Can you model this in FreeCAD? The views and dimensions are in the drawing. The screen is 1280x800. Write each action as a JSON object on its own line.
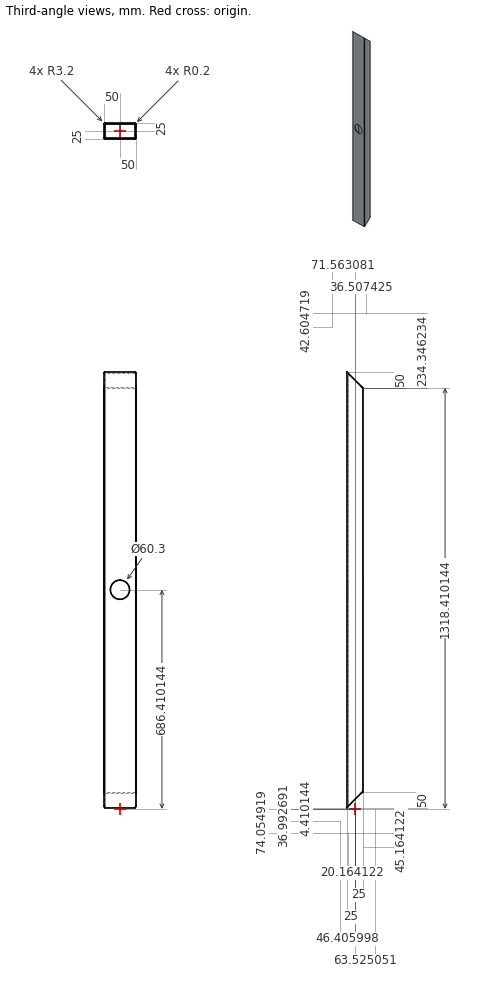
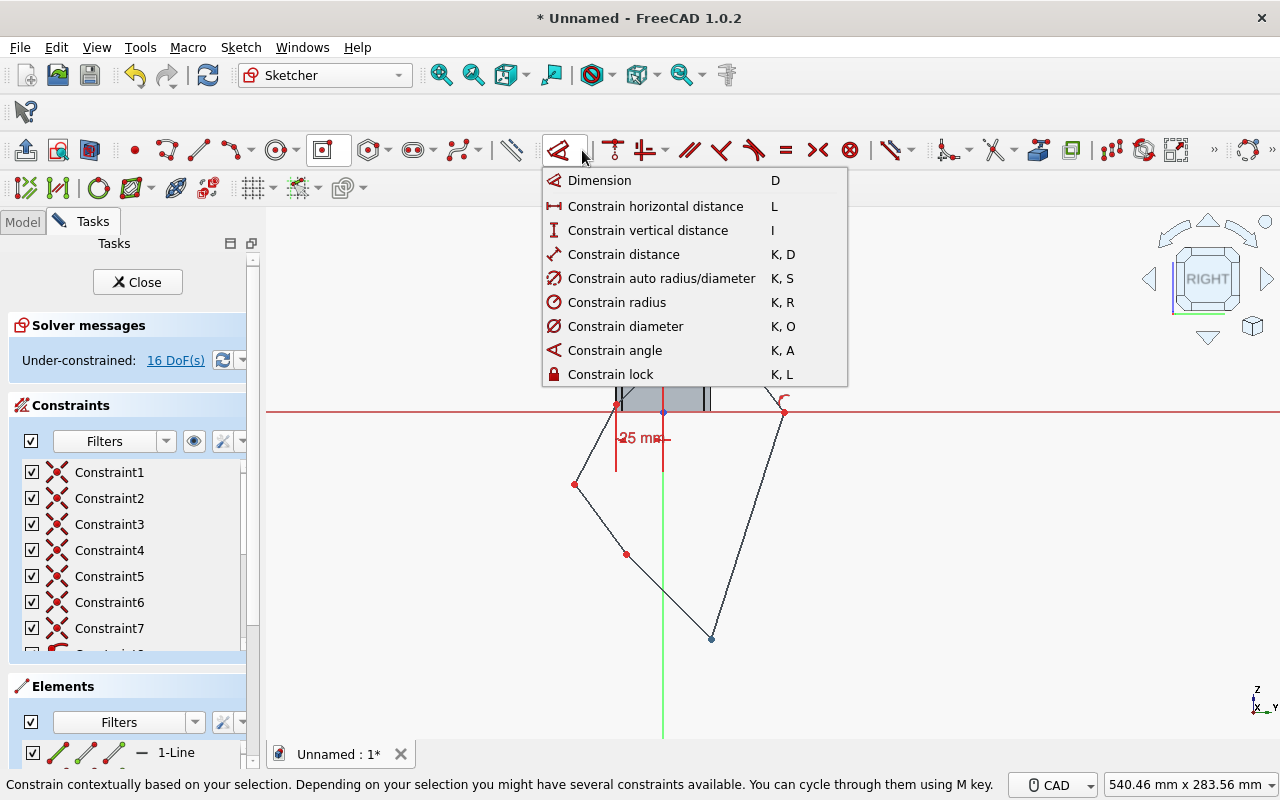
{"action": "left_click", "coordinate": [695, 206]}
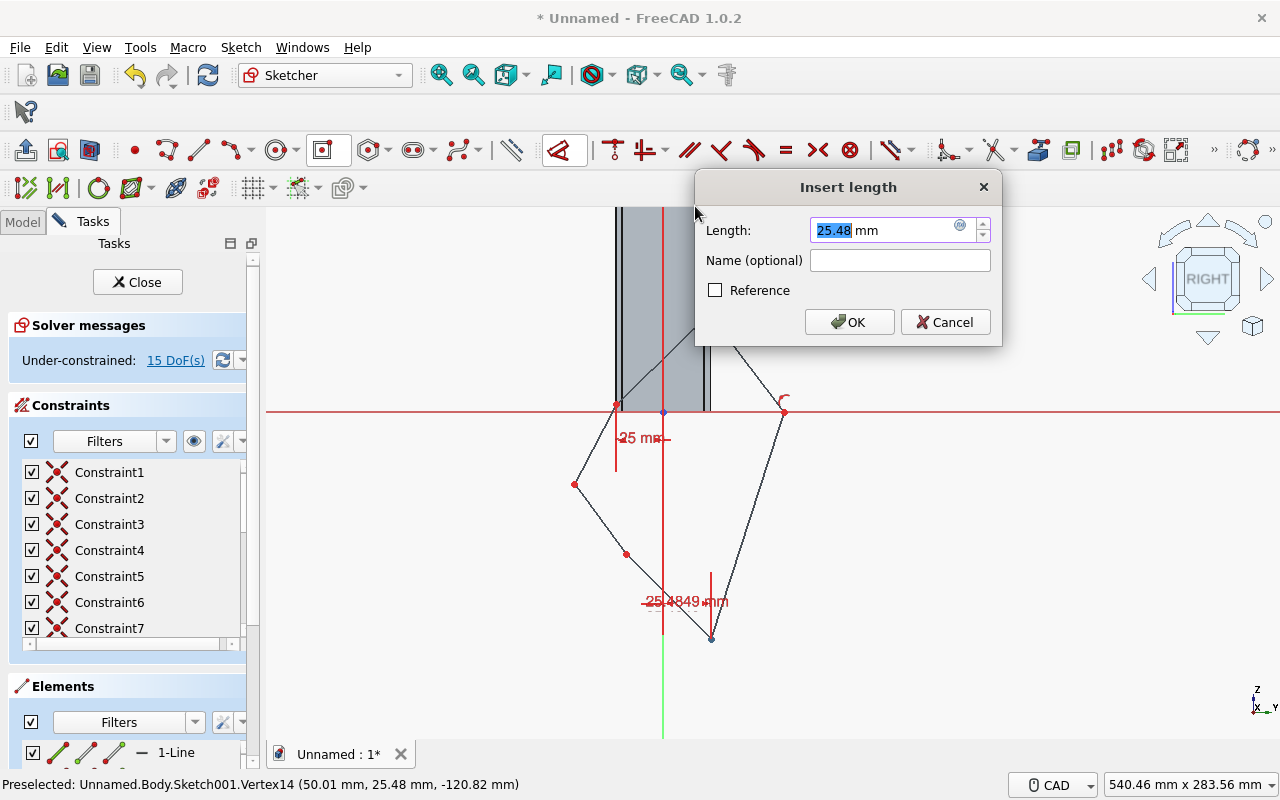
{"action": "type", "text": "25"}
{"action": "key", "text": "Return"}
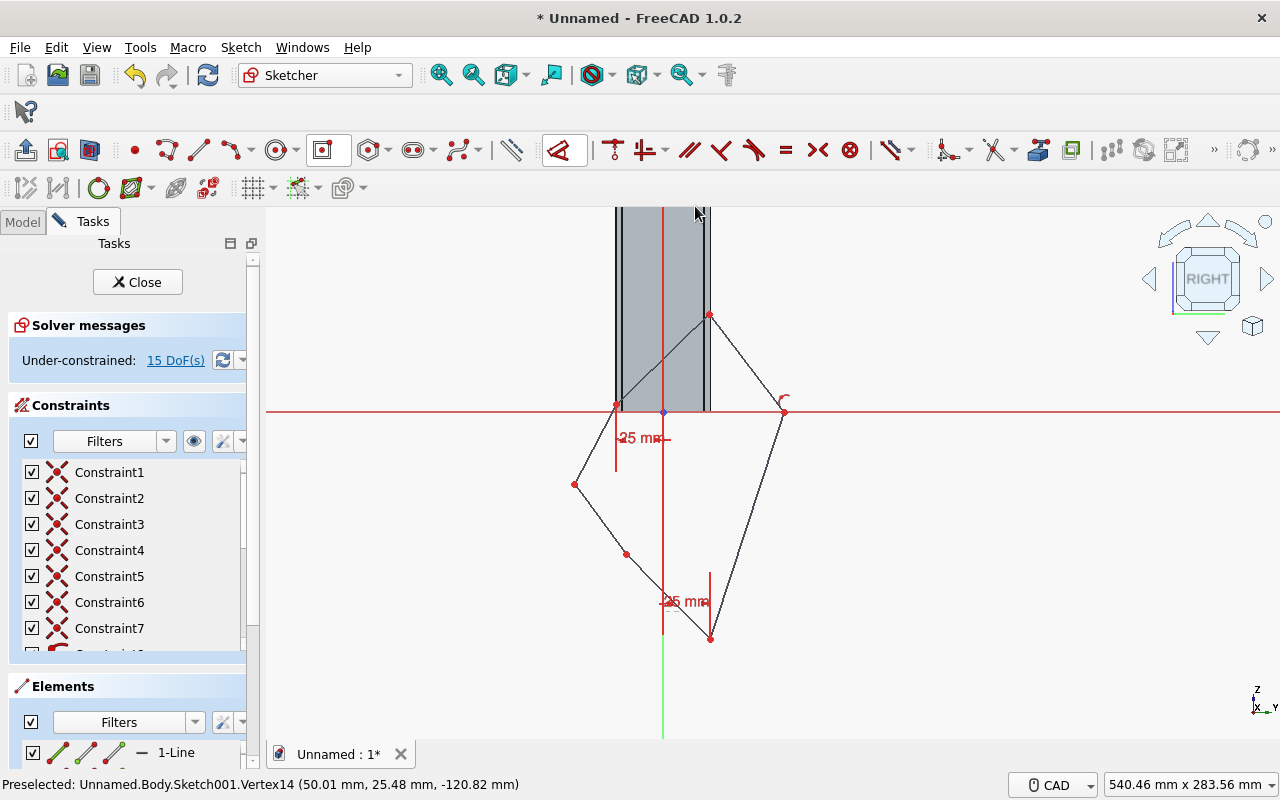
{"action": "left_click", "coordinate": [709, 314]}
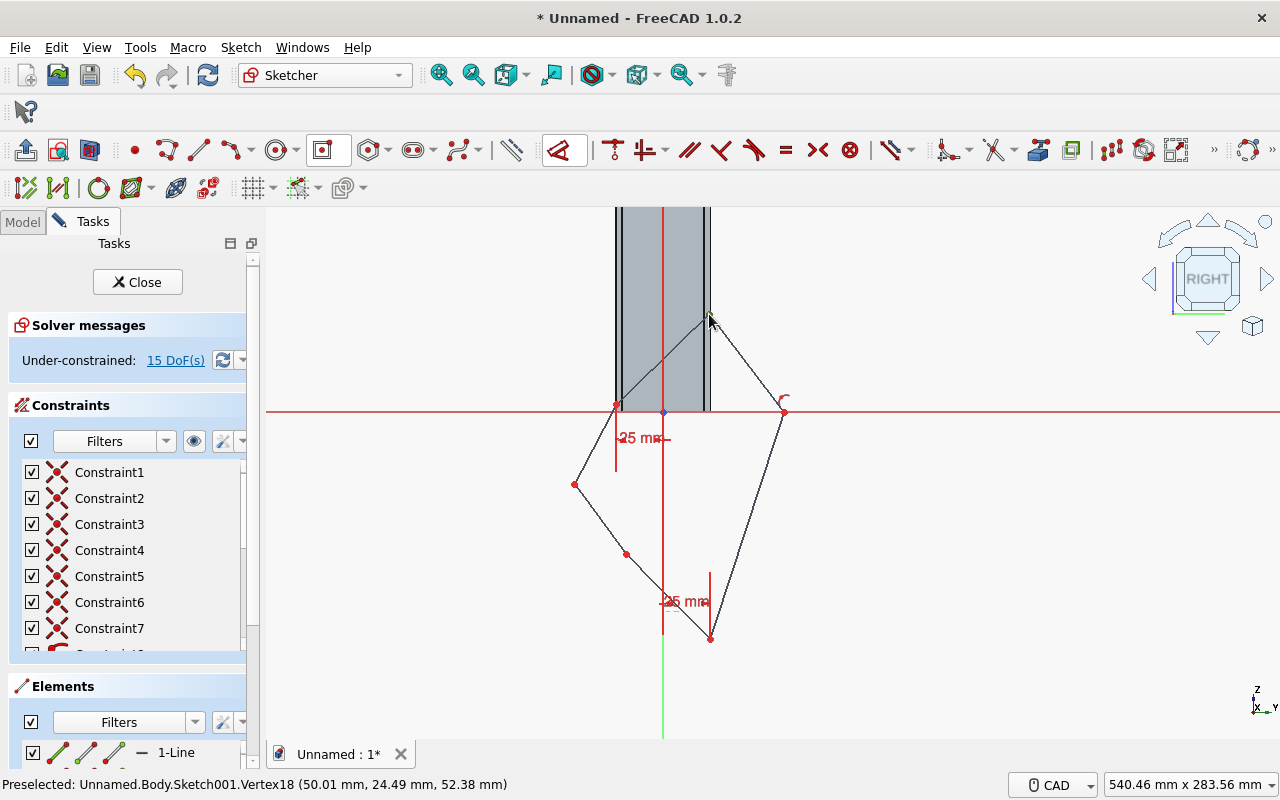
{"action": "left_click", "coordinate": [582, 150]}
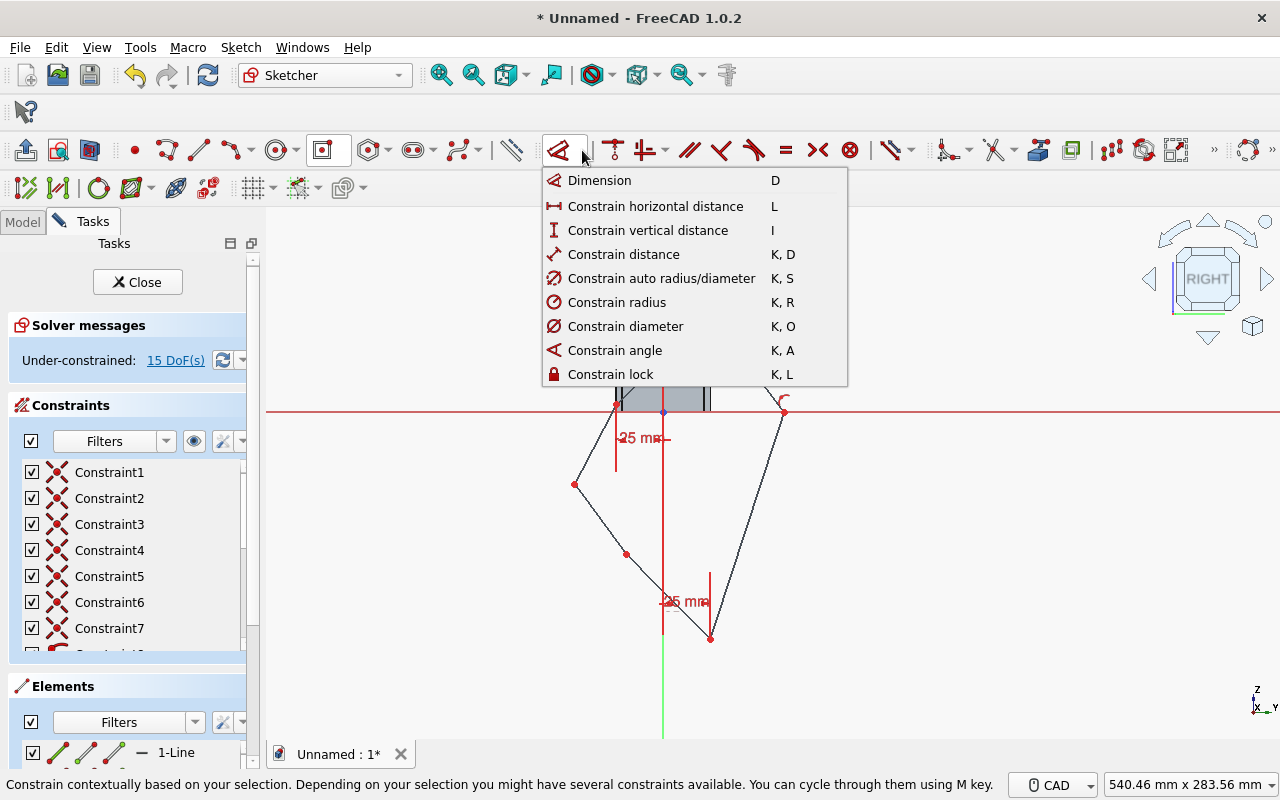
{"action": "left_click", "coordinate": [695, 206]}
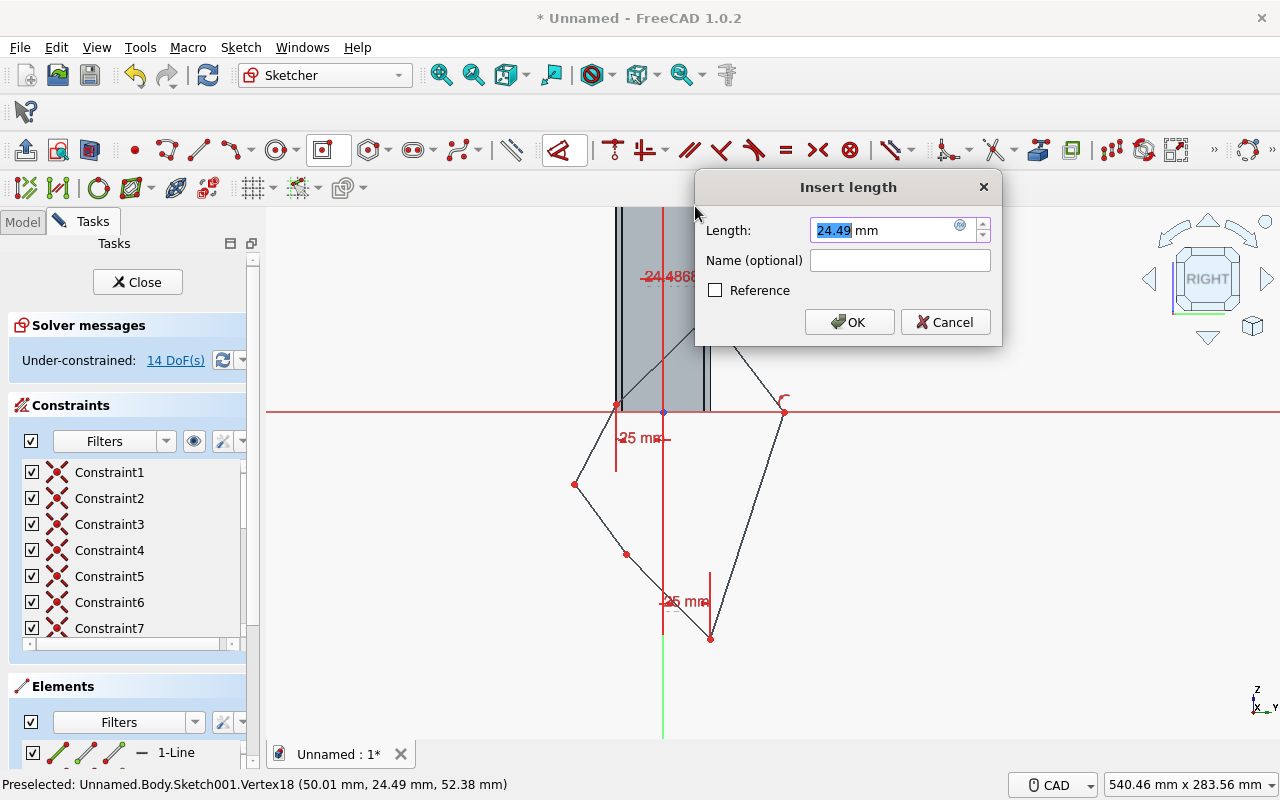
{"action": "type", "text": "25"}
{"action": "key", "text": "Return"}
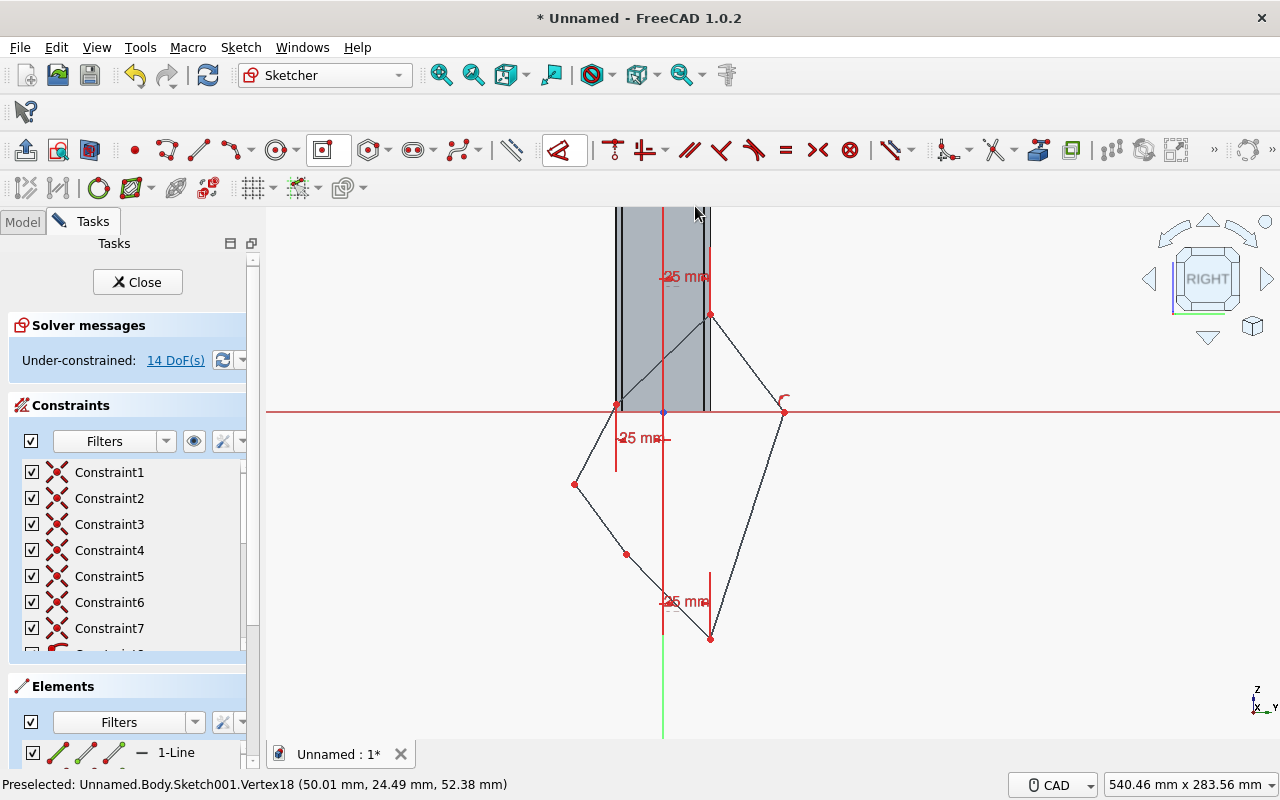
{"action": "scroll", "coordinate": [711, 648], "scroll_direction": "down", "scroll_amount": 11}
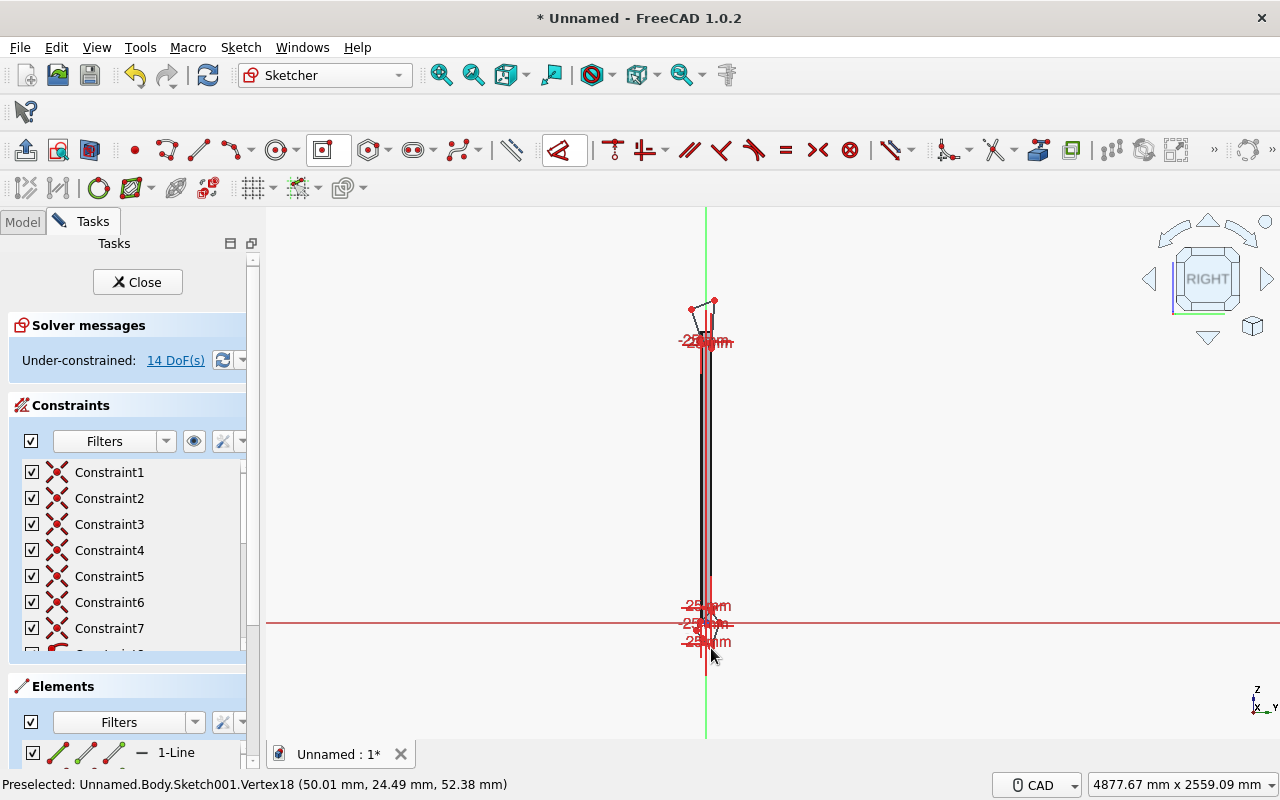
{"action": "scroll", "coordinate": [704, 342], "scroll_direction": "up", "scroll_amount": 10}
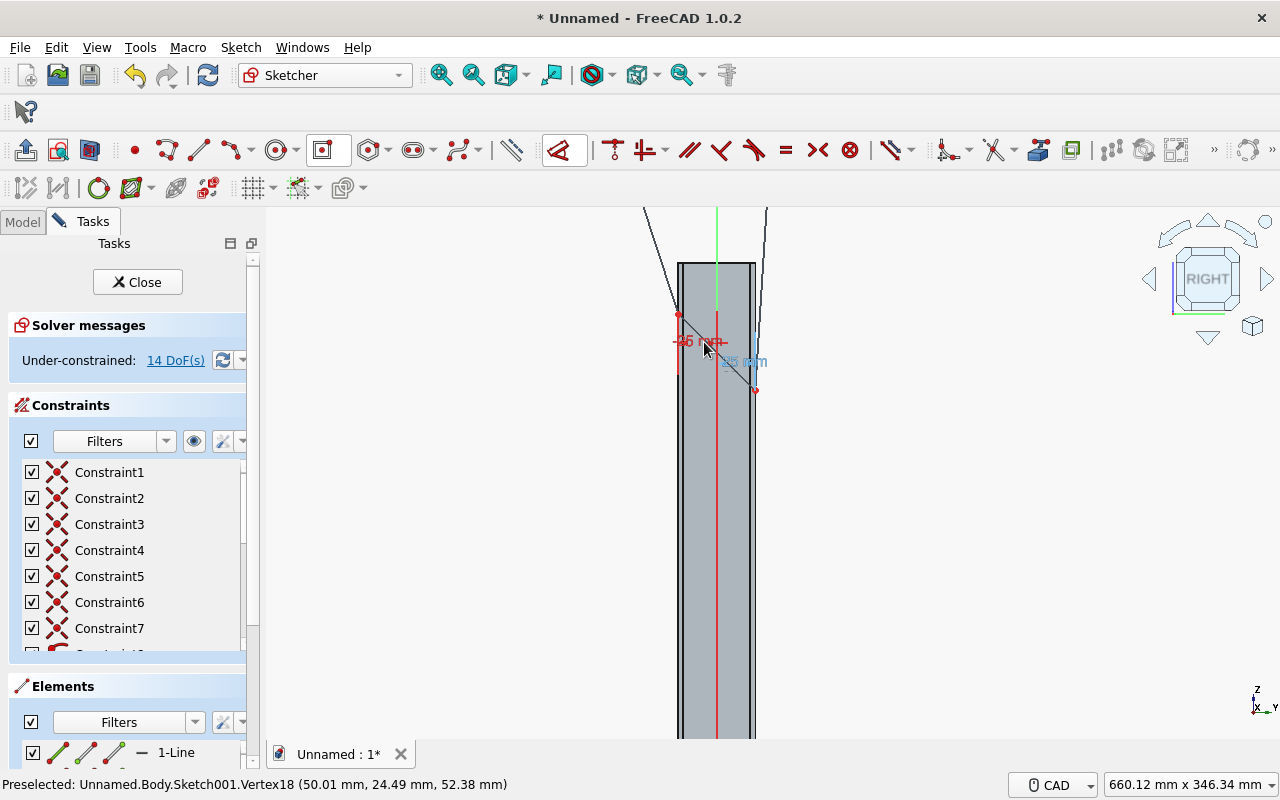
{"action": "left_click", "coordinate": [694, 329]}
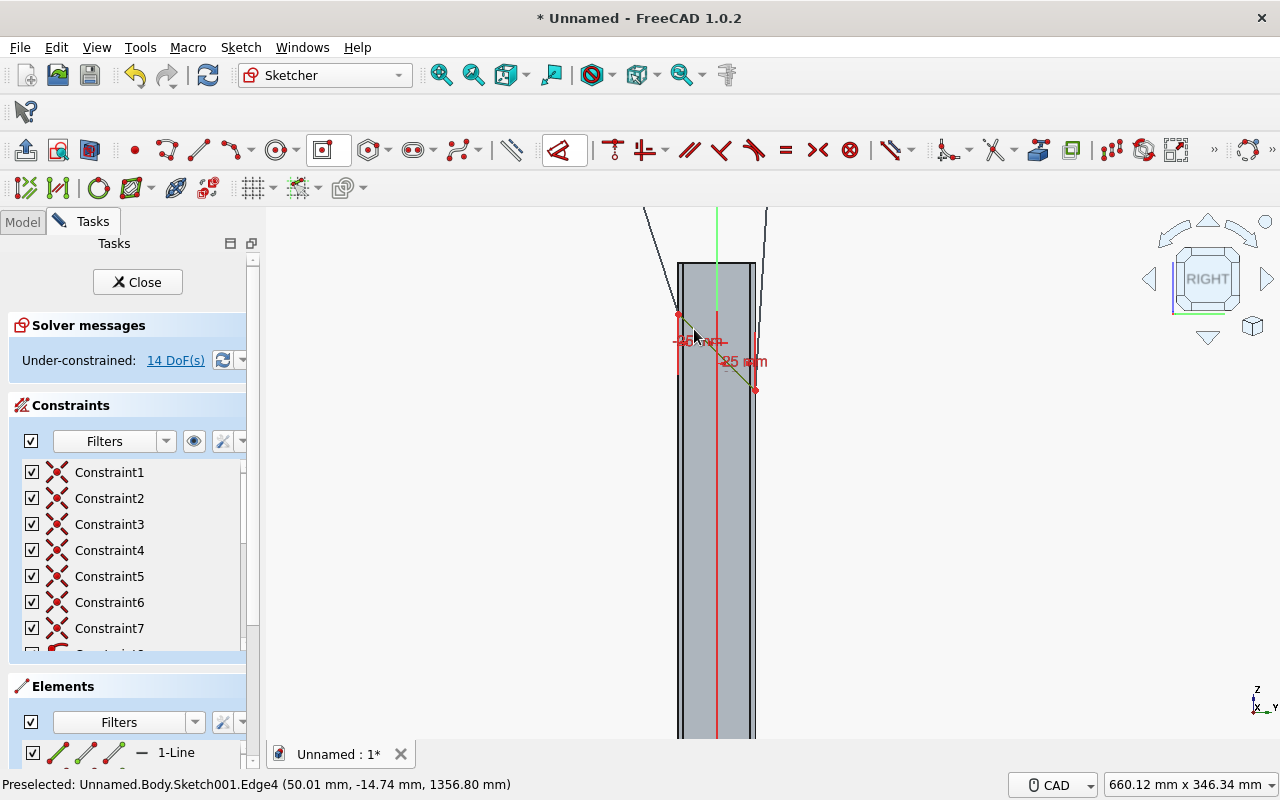
{"action": "left_click", "coordinate": [582, 150]}